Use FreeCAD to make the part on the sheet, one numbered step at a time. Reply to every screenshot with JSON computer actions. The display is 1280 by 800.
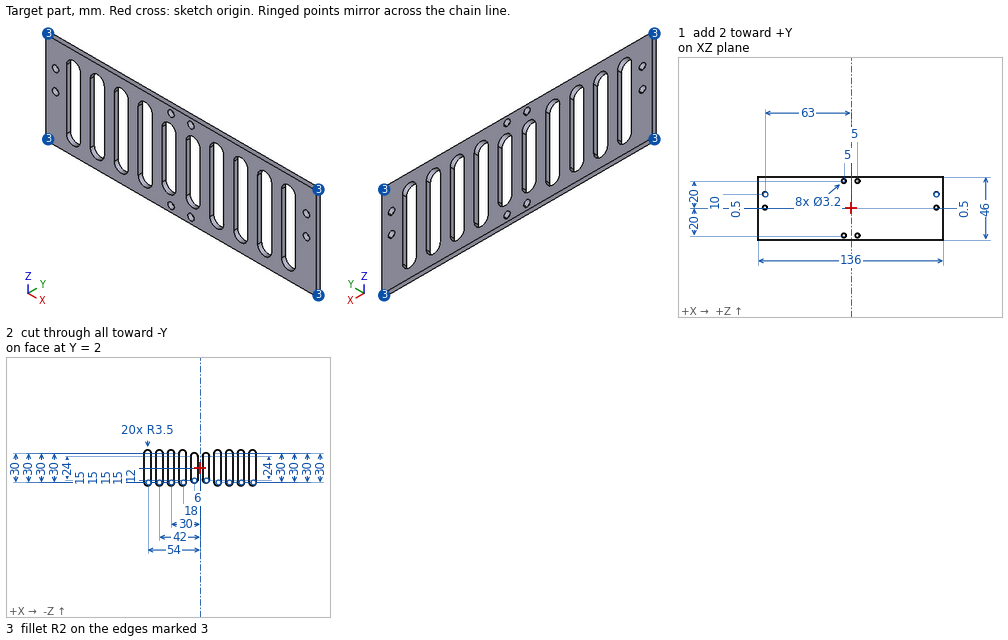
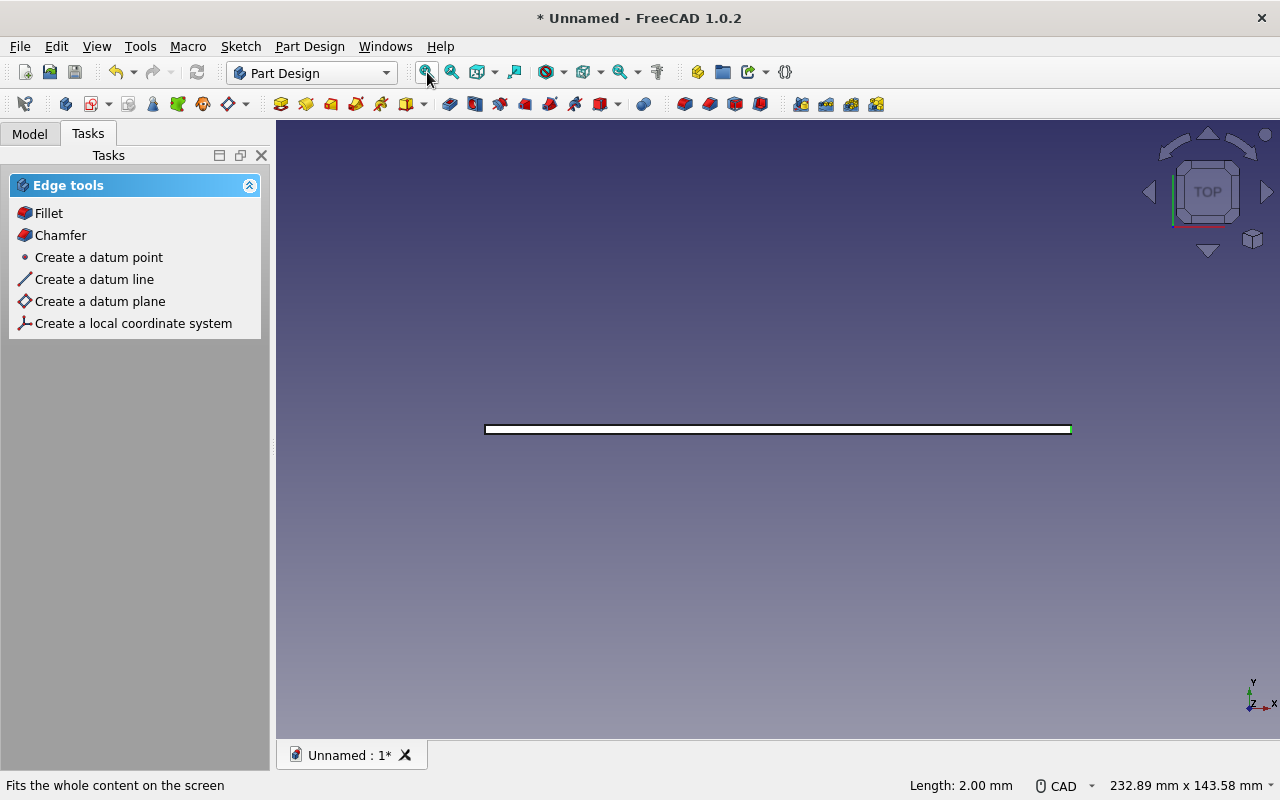
{"action": "scroll", "coordinate": [485, 428], "scroll_direction": "up", "scroll_amount": 8}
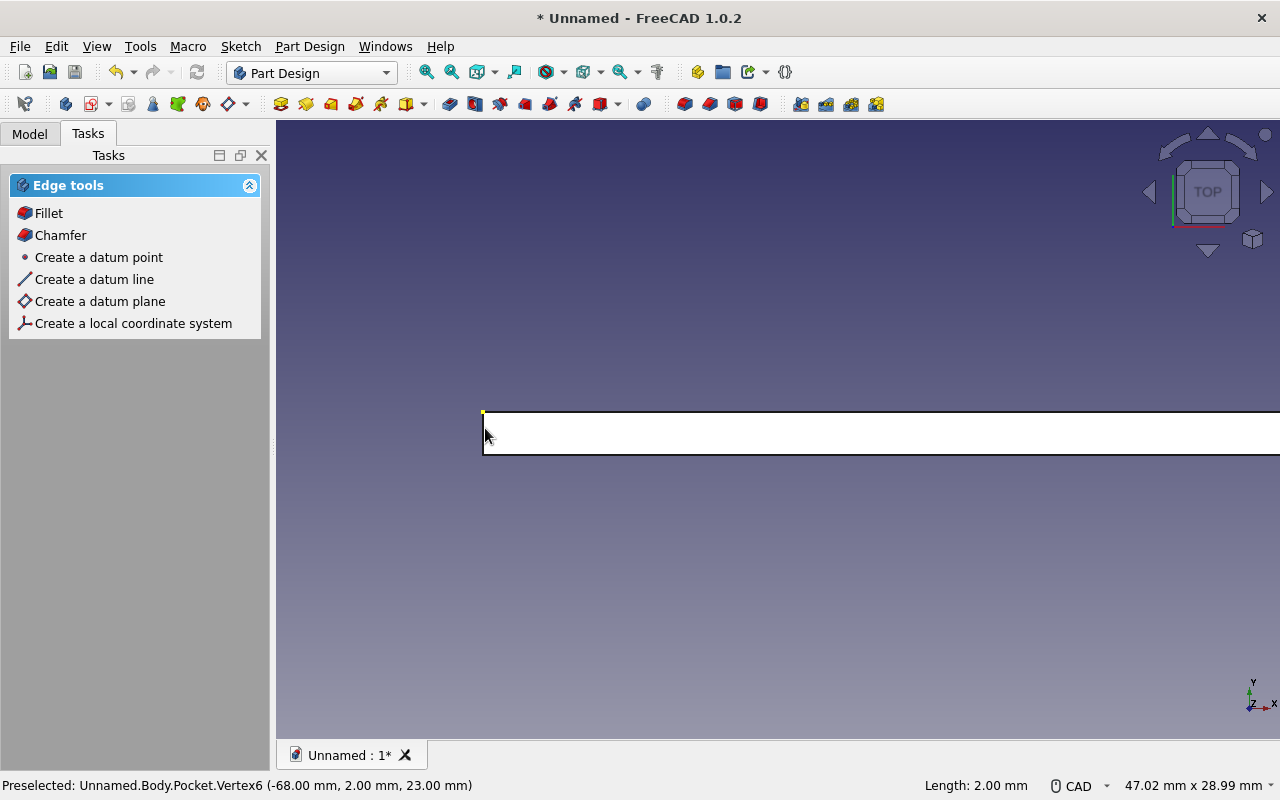
{"action": "left_click", "coordinate": [483, 432], "text": "ctrl"}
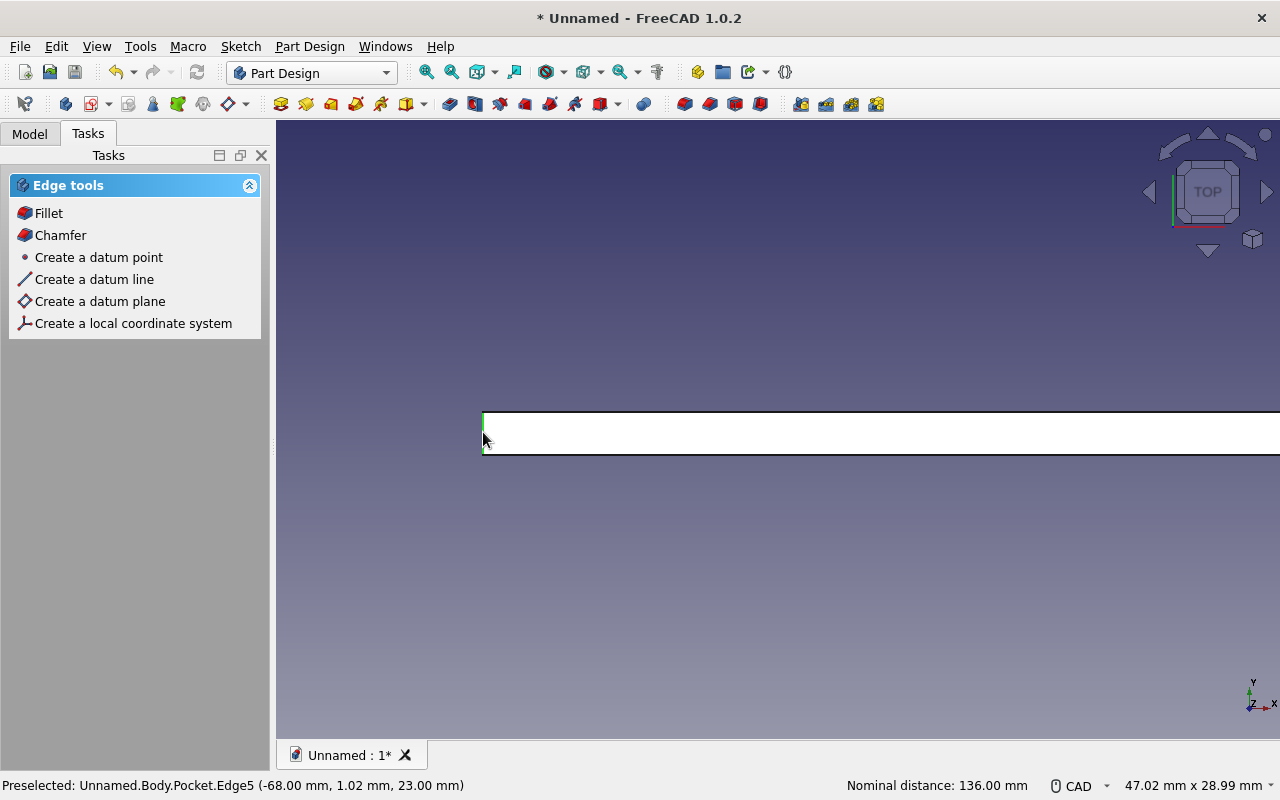
{"action": "left_click", "coordinate": [427, 72]}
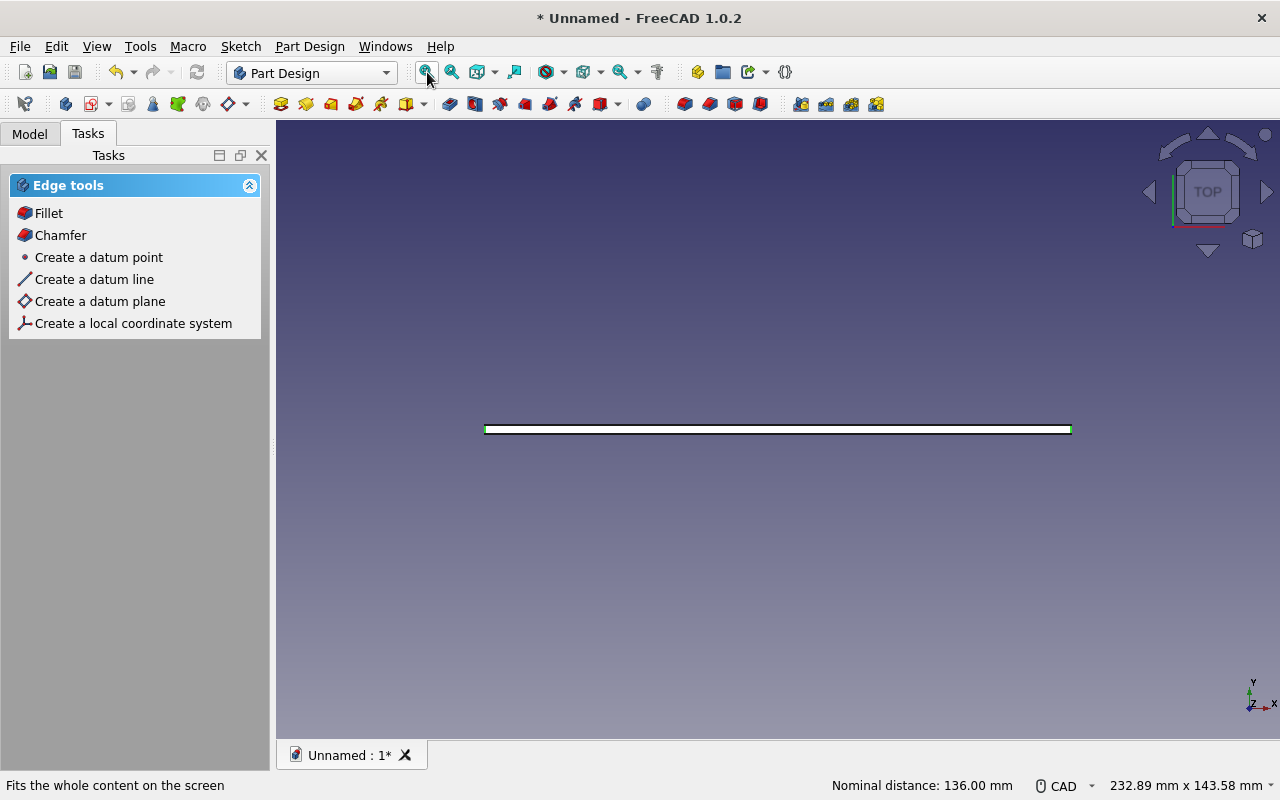
{"action": "key", "text": "1"}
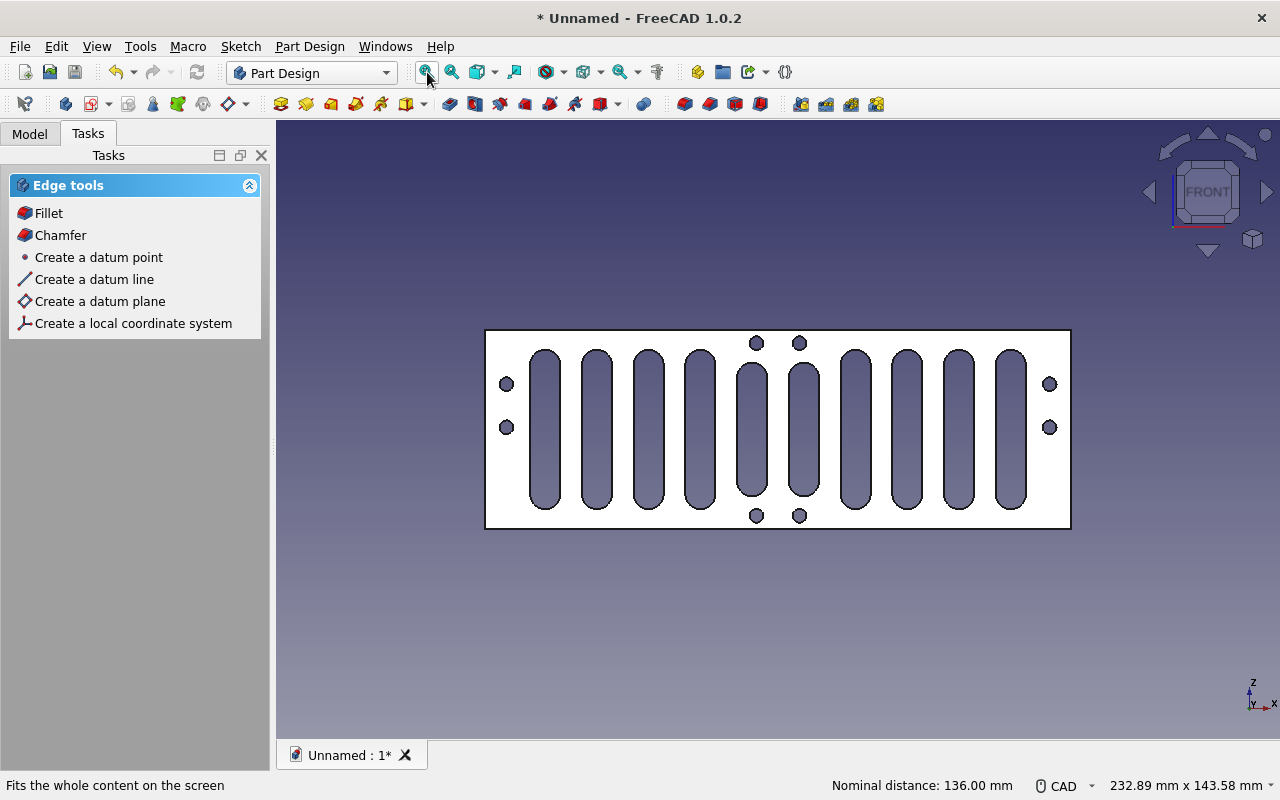
{"action": "scroll", "coordinate": [485, 528], "scroll_direction": "up", "scroll_amount": 8}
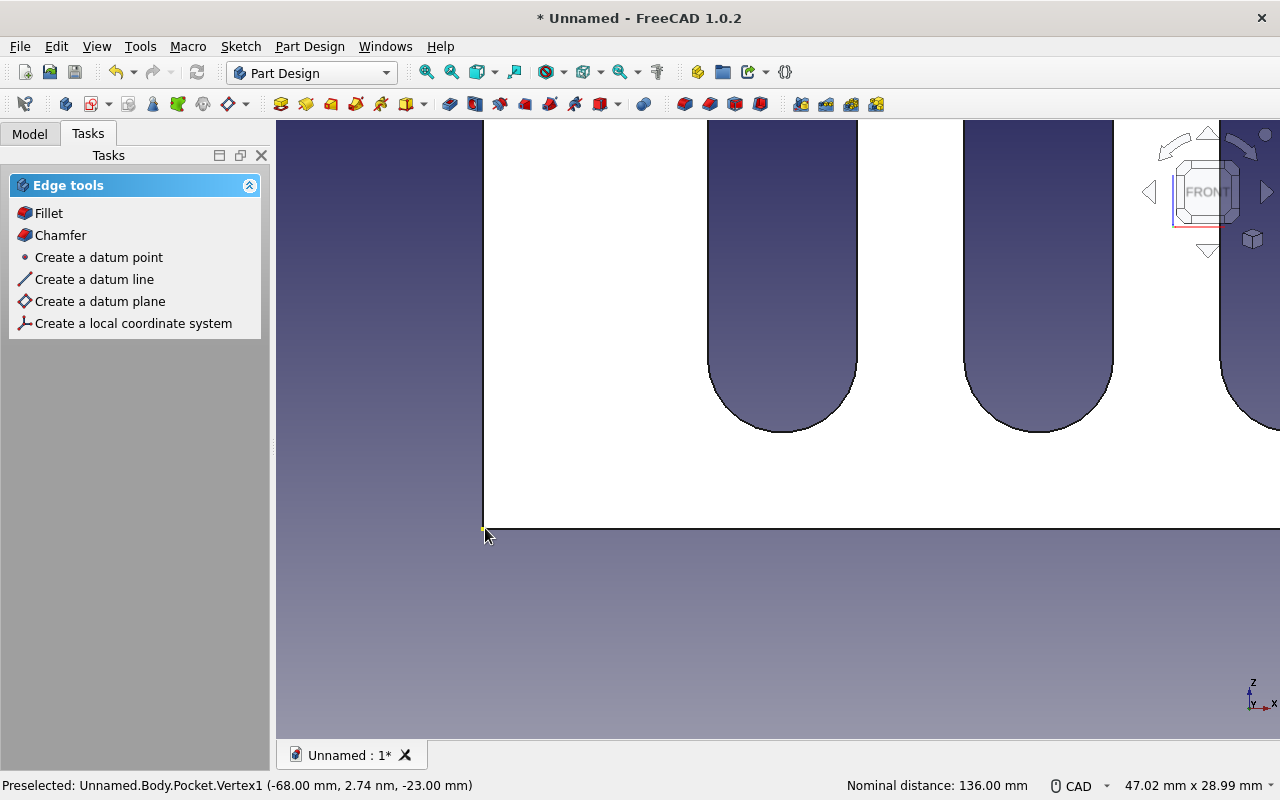
{"action": "left_click", "coordinate": [427, 72]}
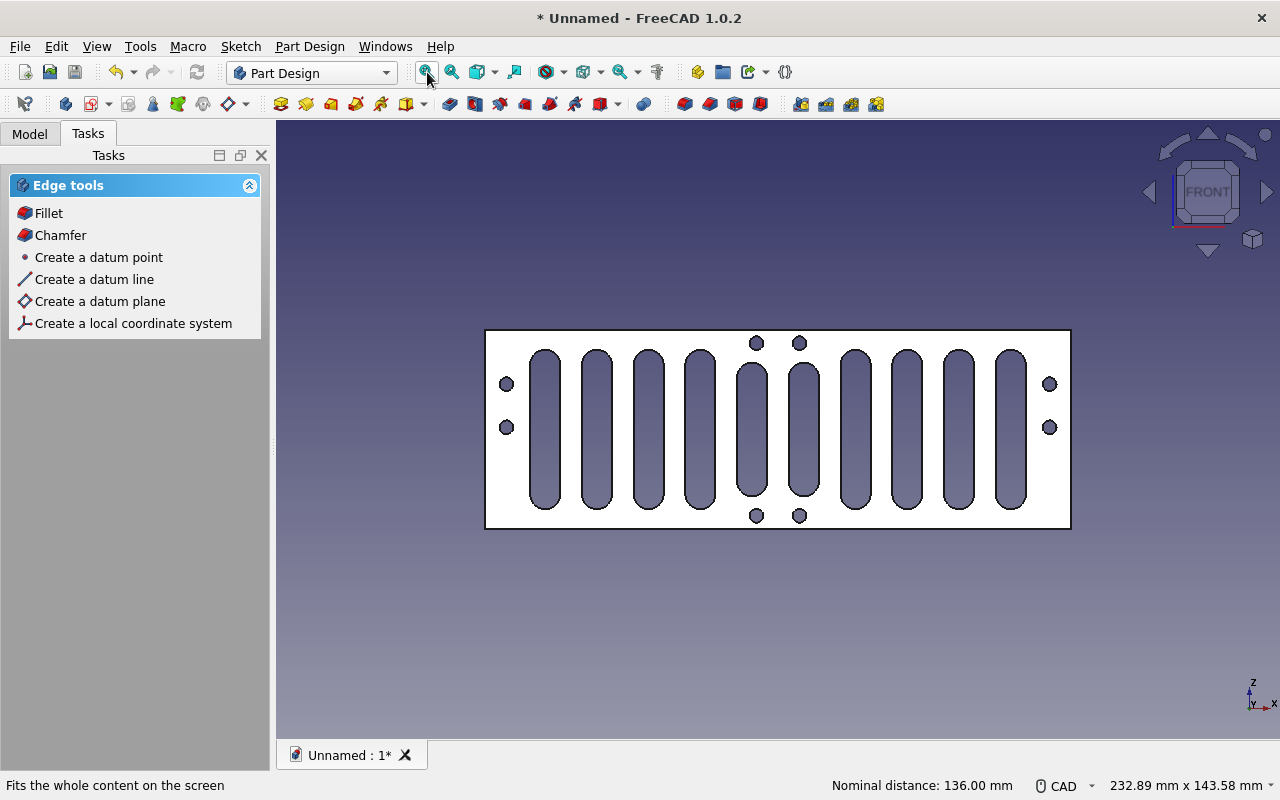
{"action": "key", "text": "3"}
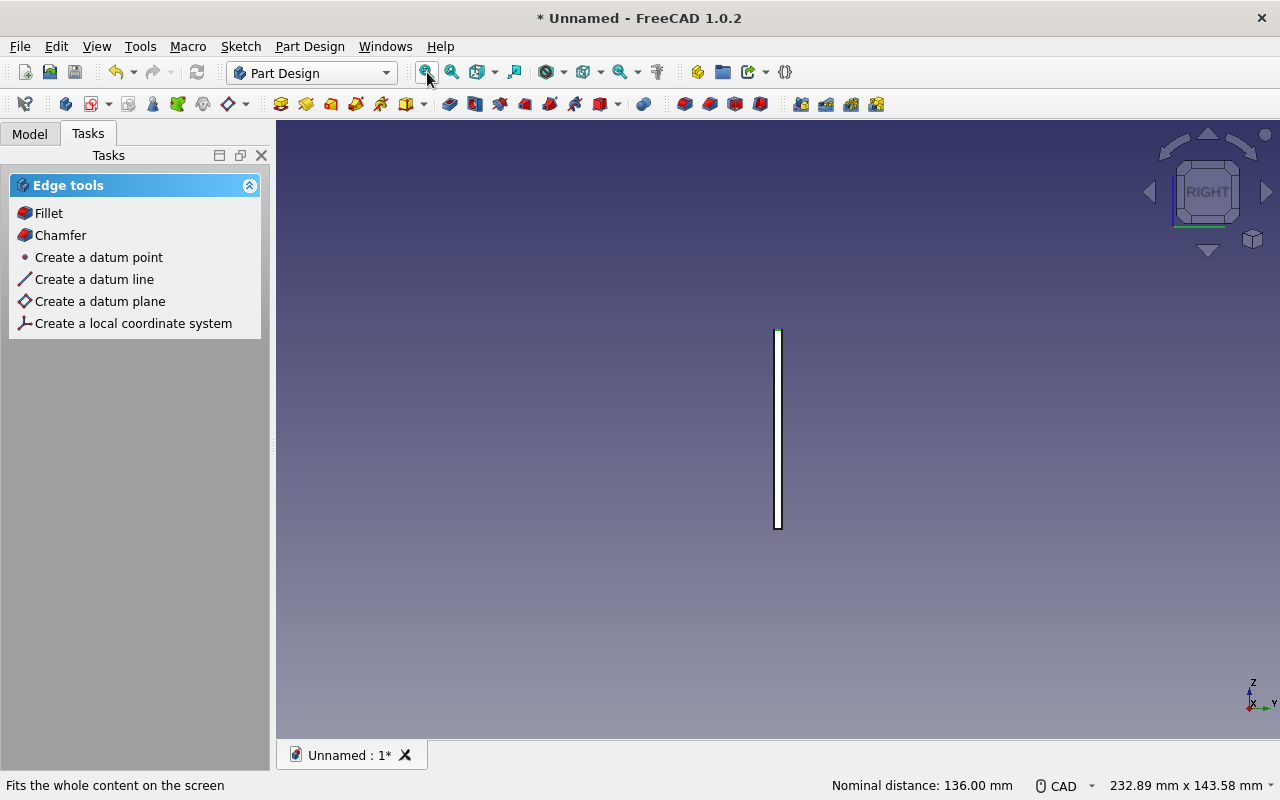
{"action": "left_click", "coordinate": [427, 72]}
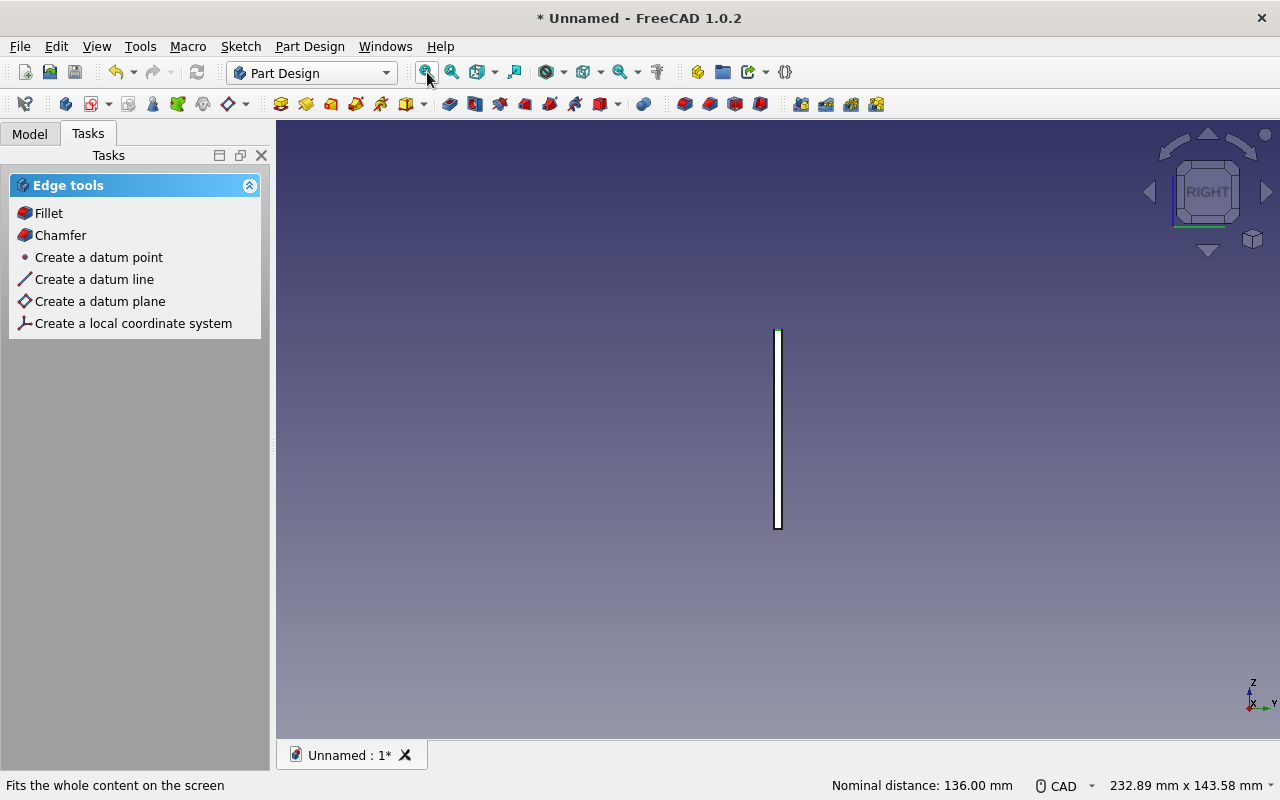
{"action": "scroll", "coordinate": [778, 528], "scroll_direction": "up", "scroll_amount": 8}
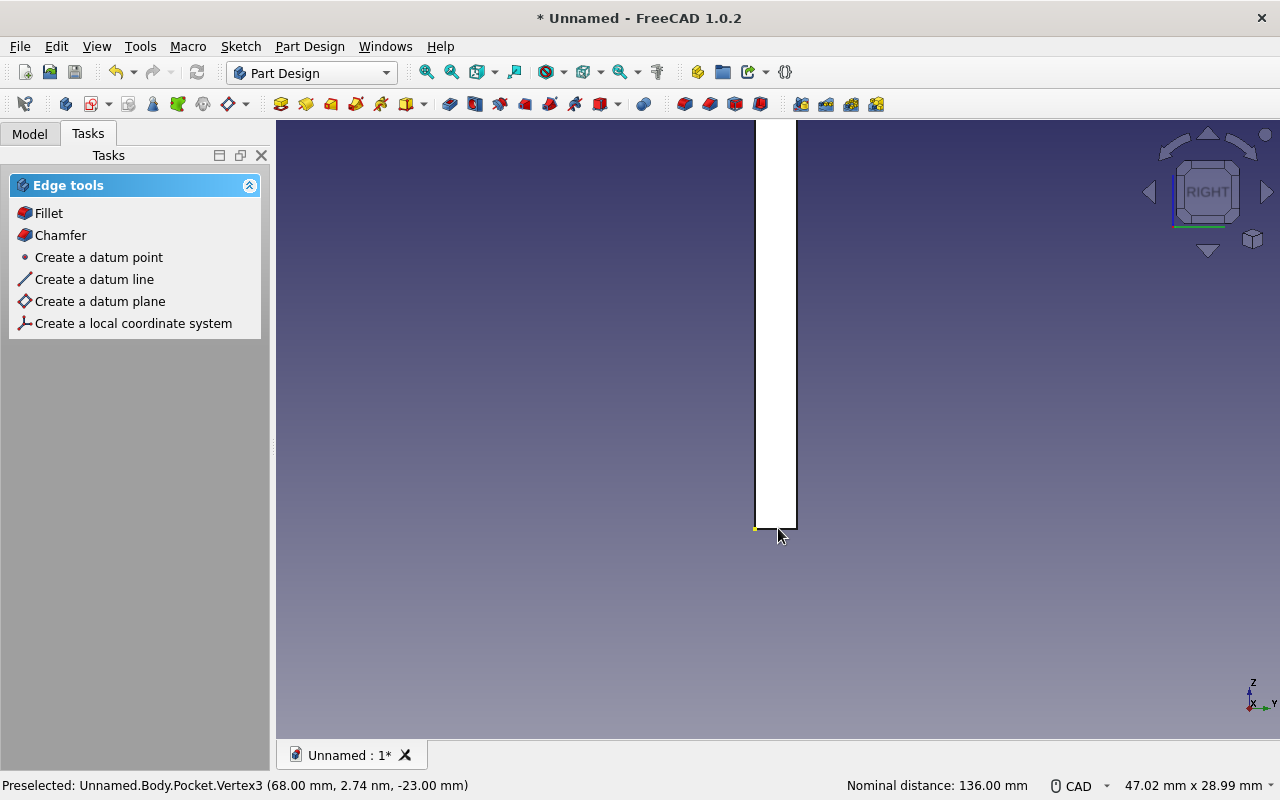
{"action": "left_click", "coordinate": [776, 528], "text": "ctrl"}